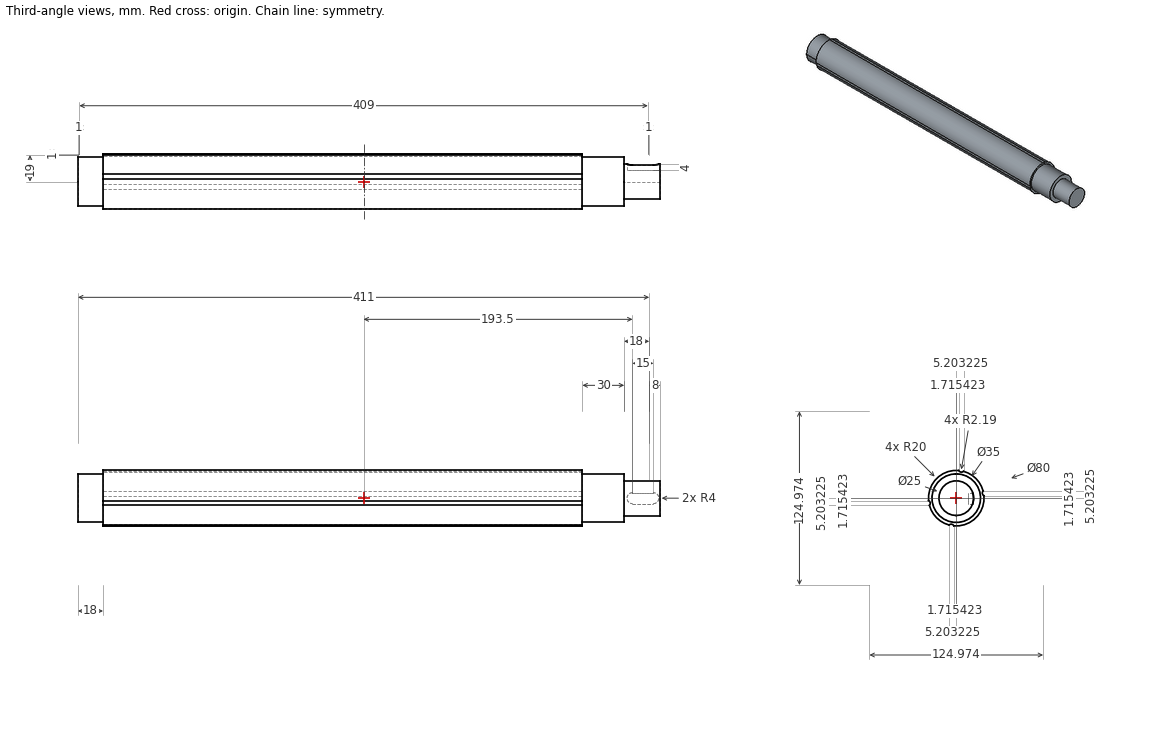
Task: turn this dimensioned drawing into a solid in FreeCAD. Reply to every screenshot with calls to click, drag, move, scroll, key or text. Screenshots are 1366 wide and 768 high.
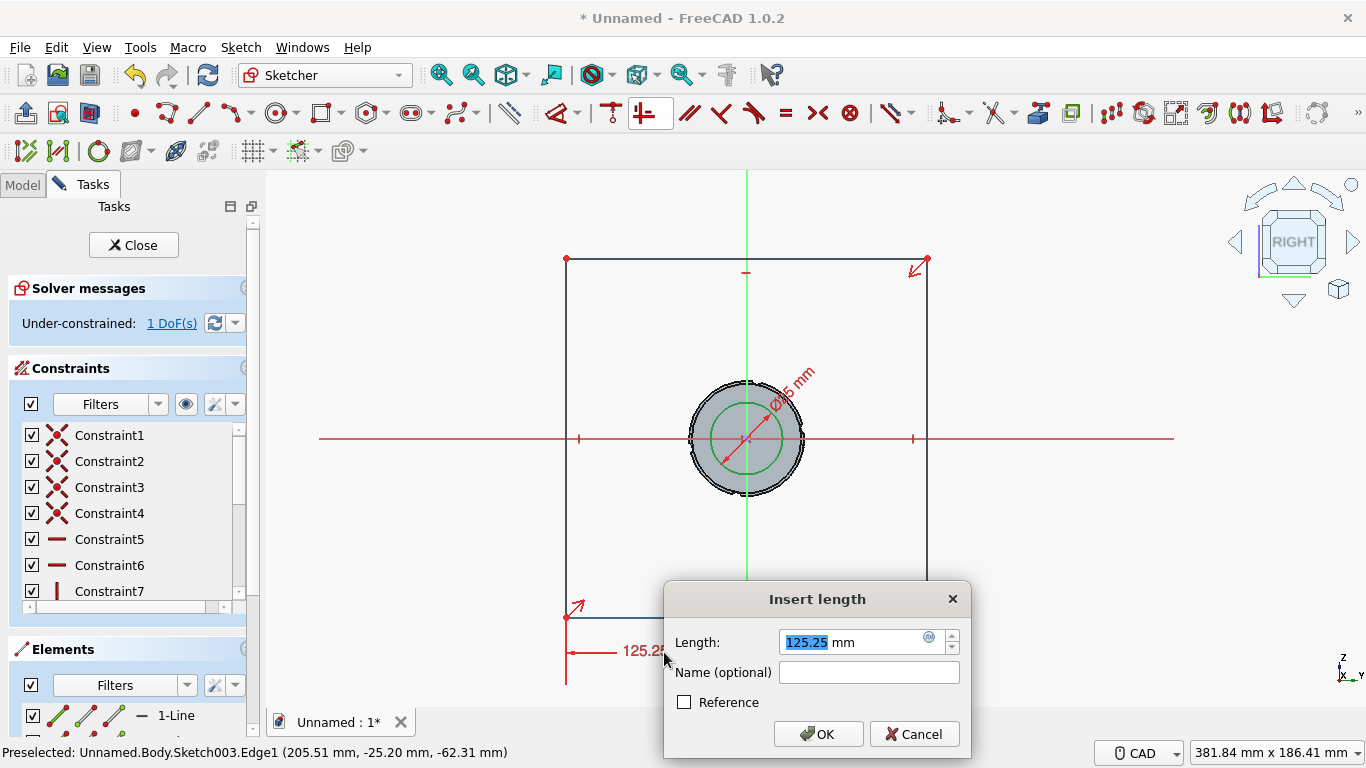
text(124.974)
key(Return)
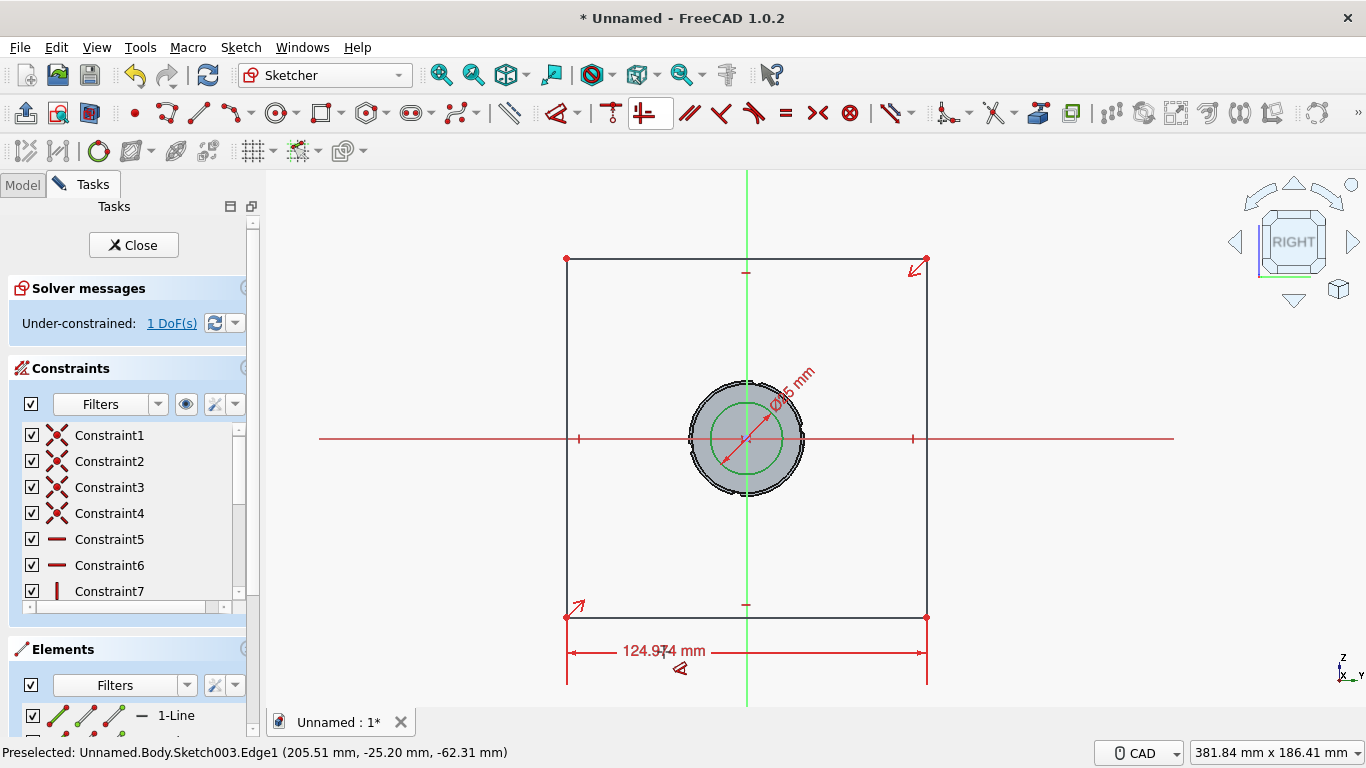
click(927, 510)
click(961, 356)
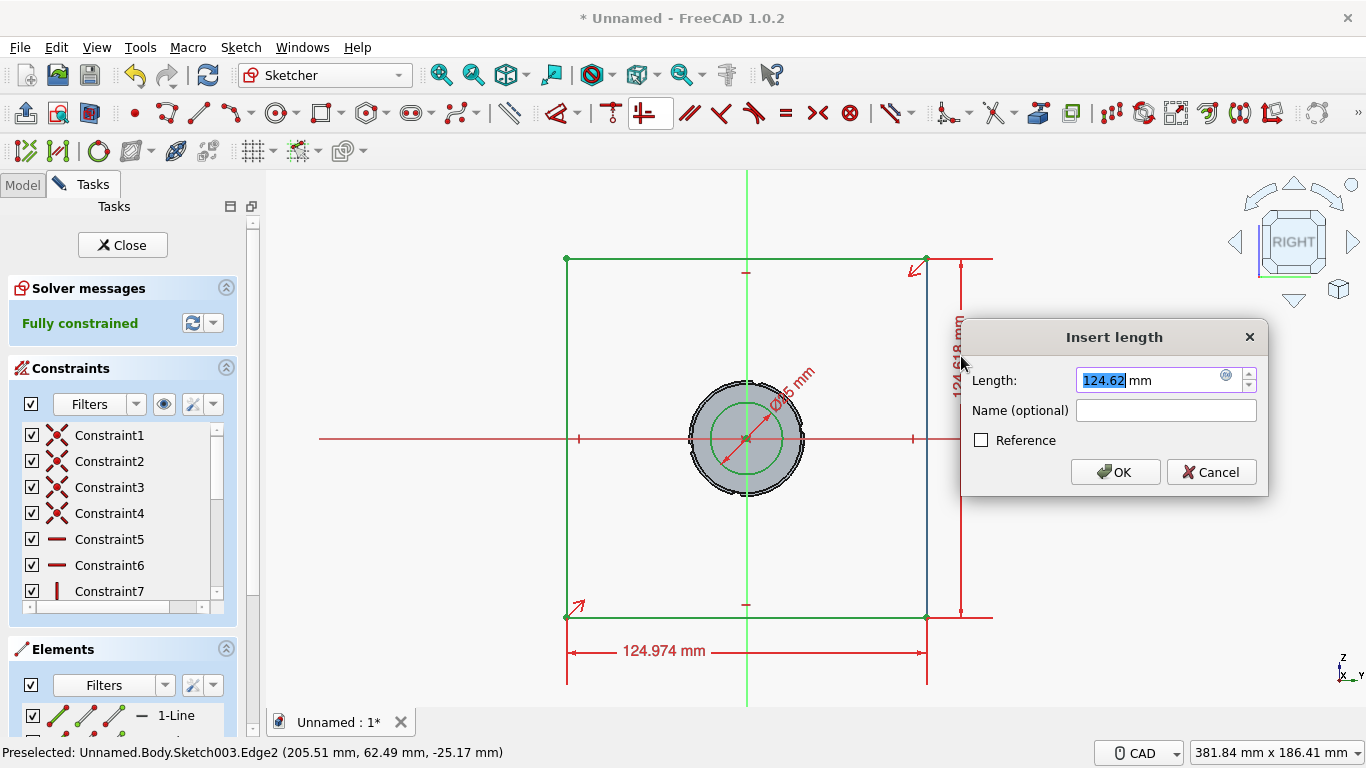
text(124.974)
key(Return)
key(Escape)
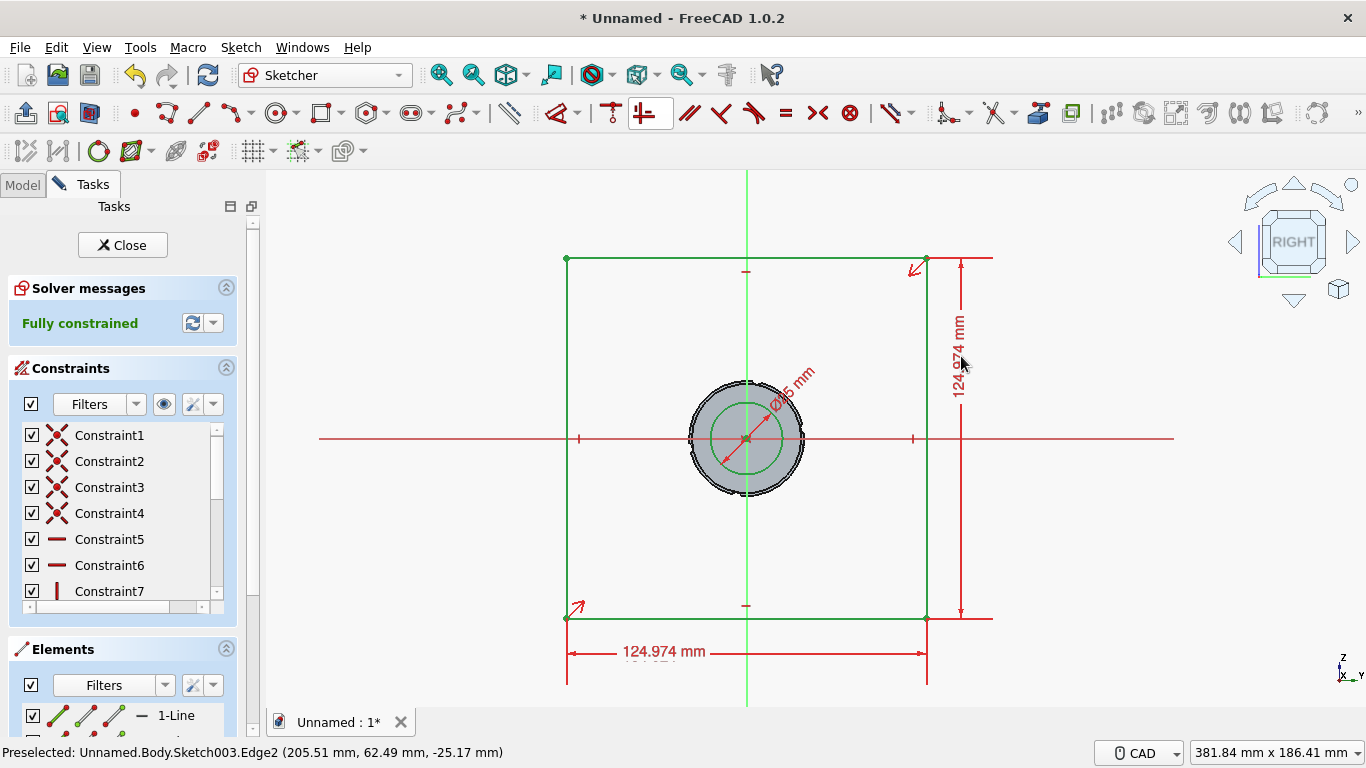
click(123, 245)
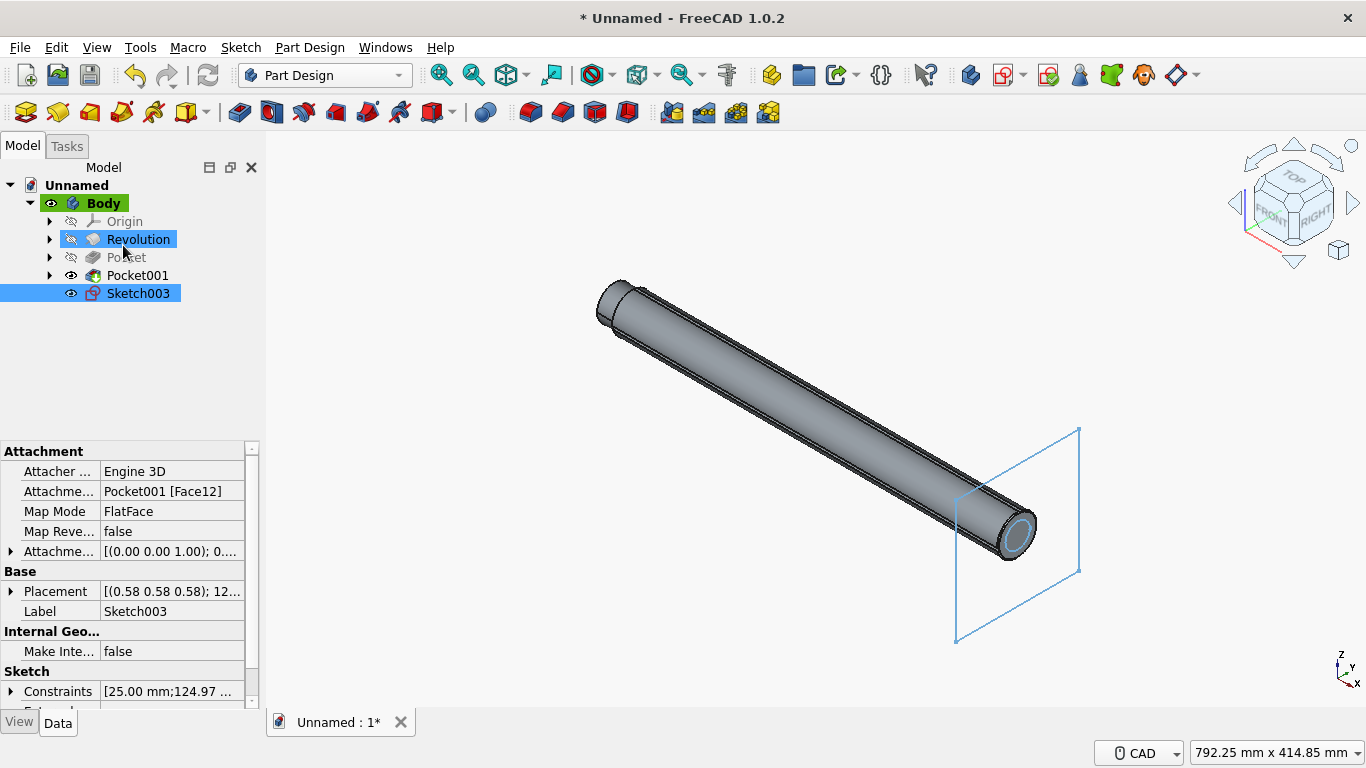
click(240, 112)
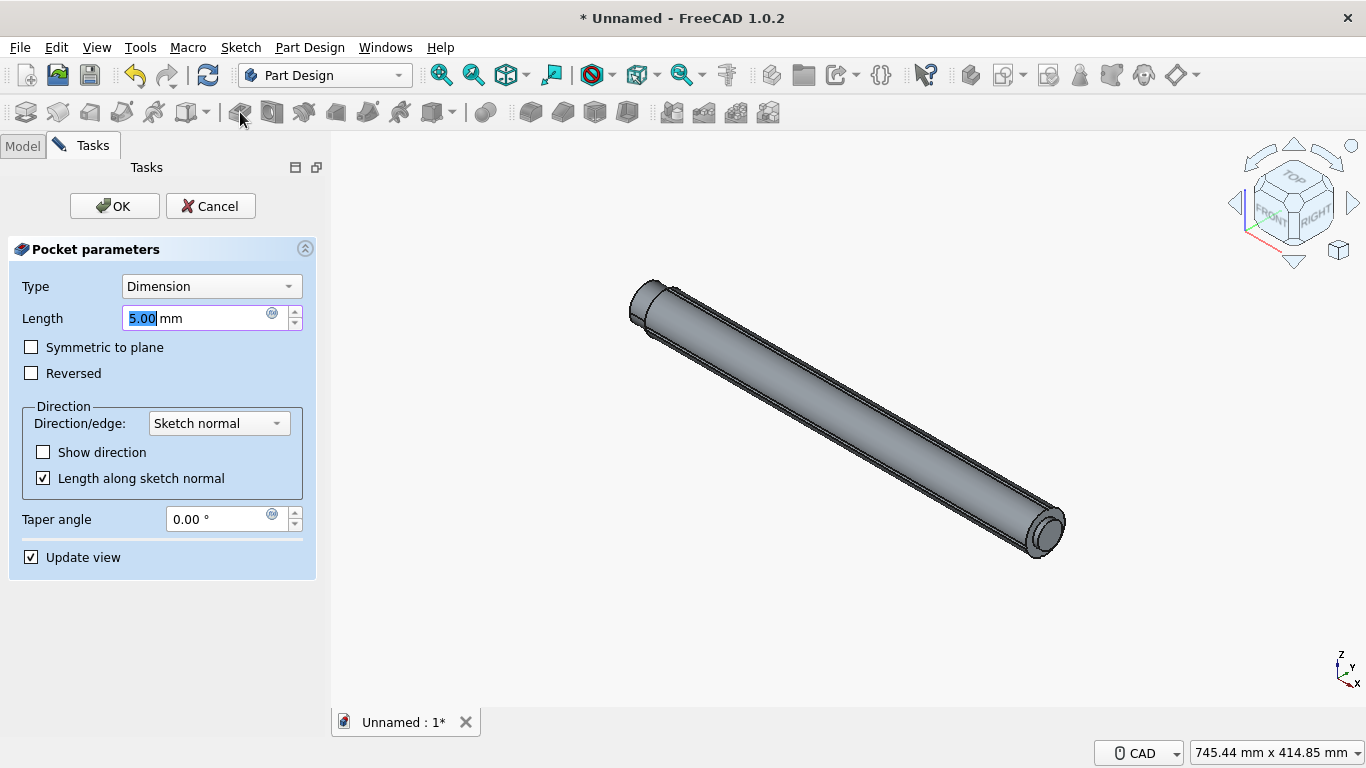
text(18)
key(Tab)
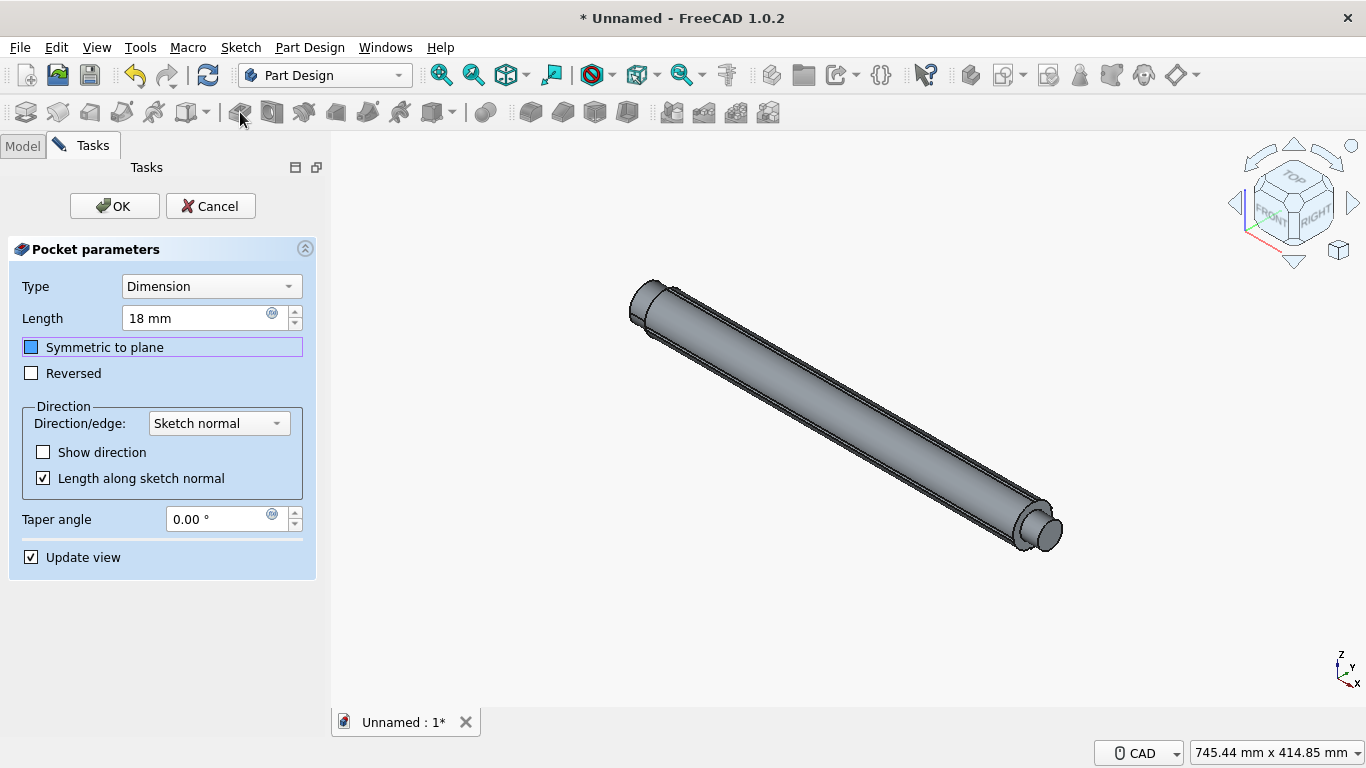
click(115, 206)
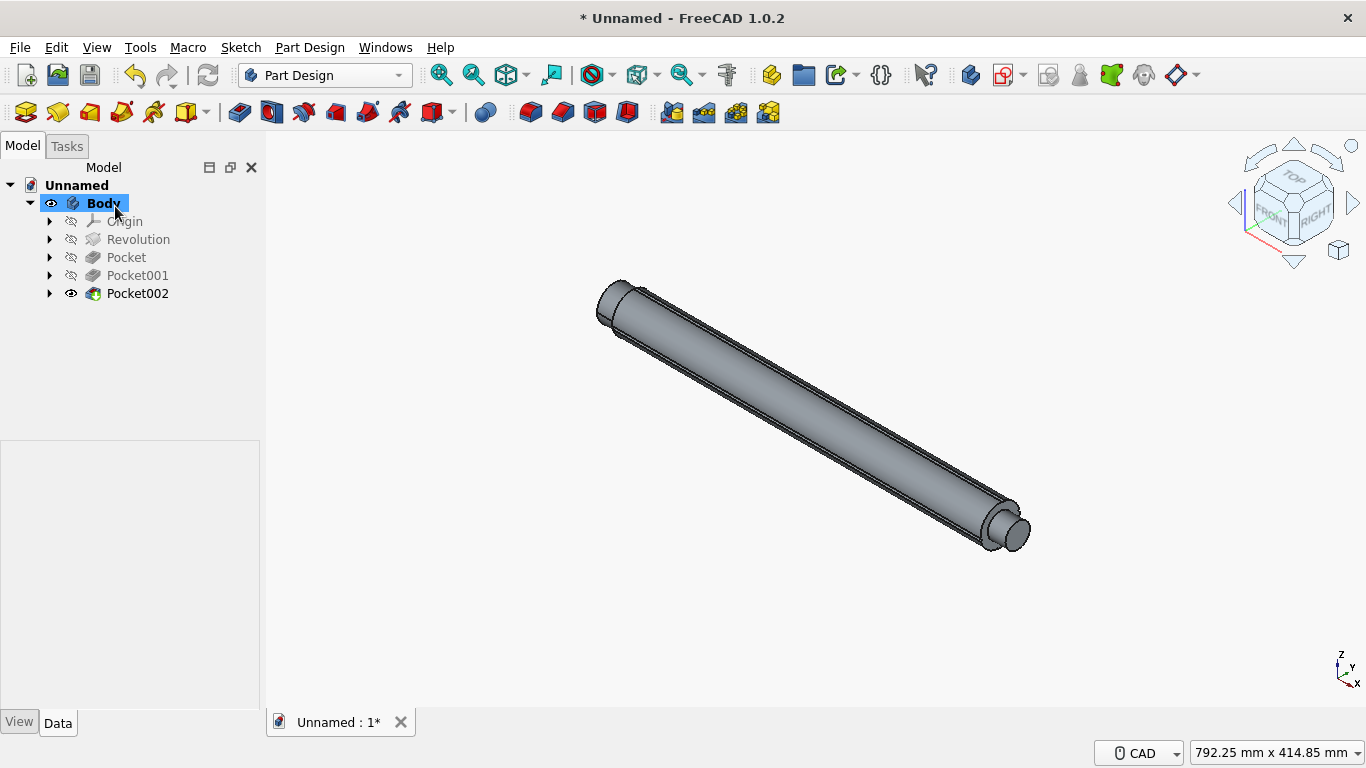
scroll(989, 518, up, 5)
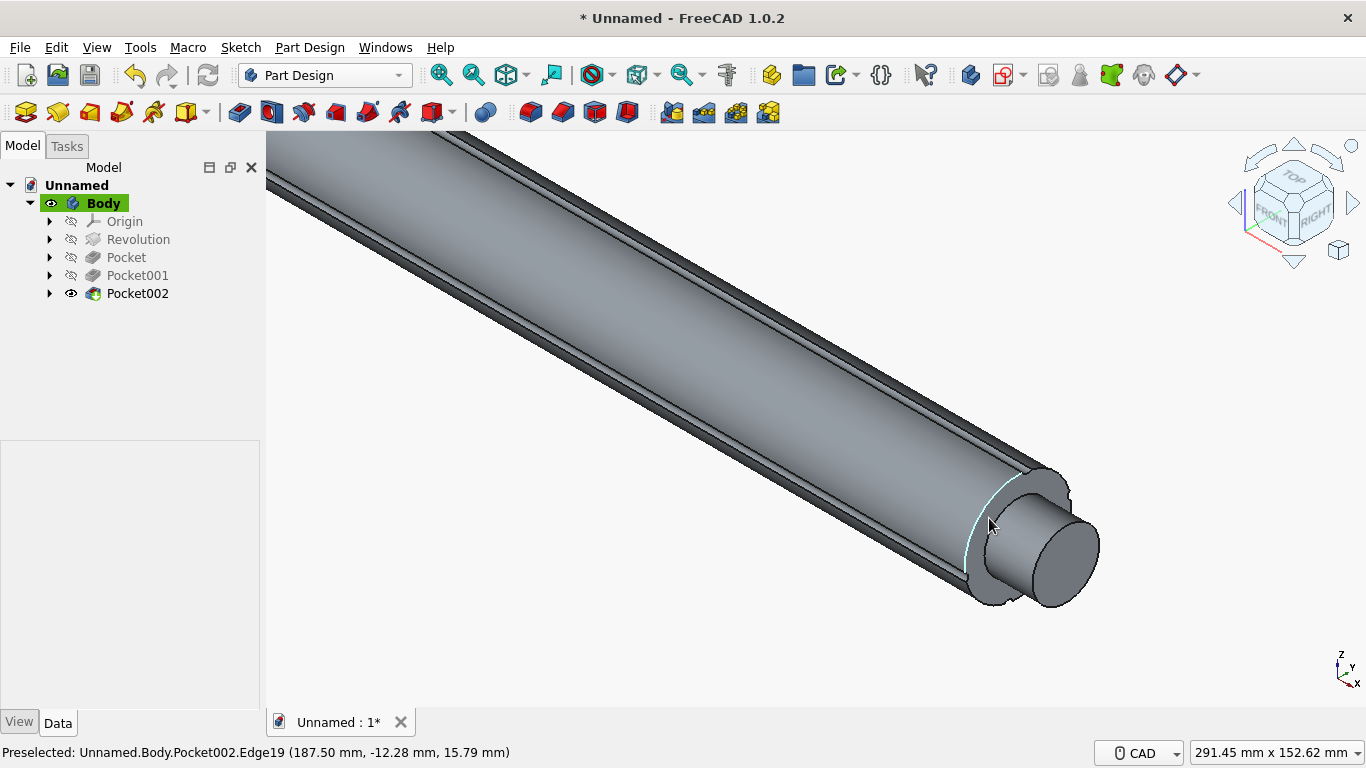
click(1048, 483)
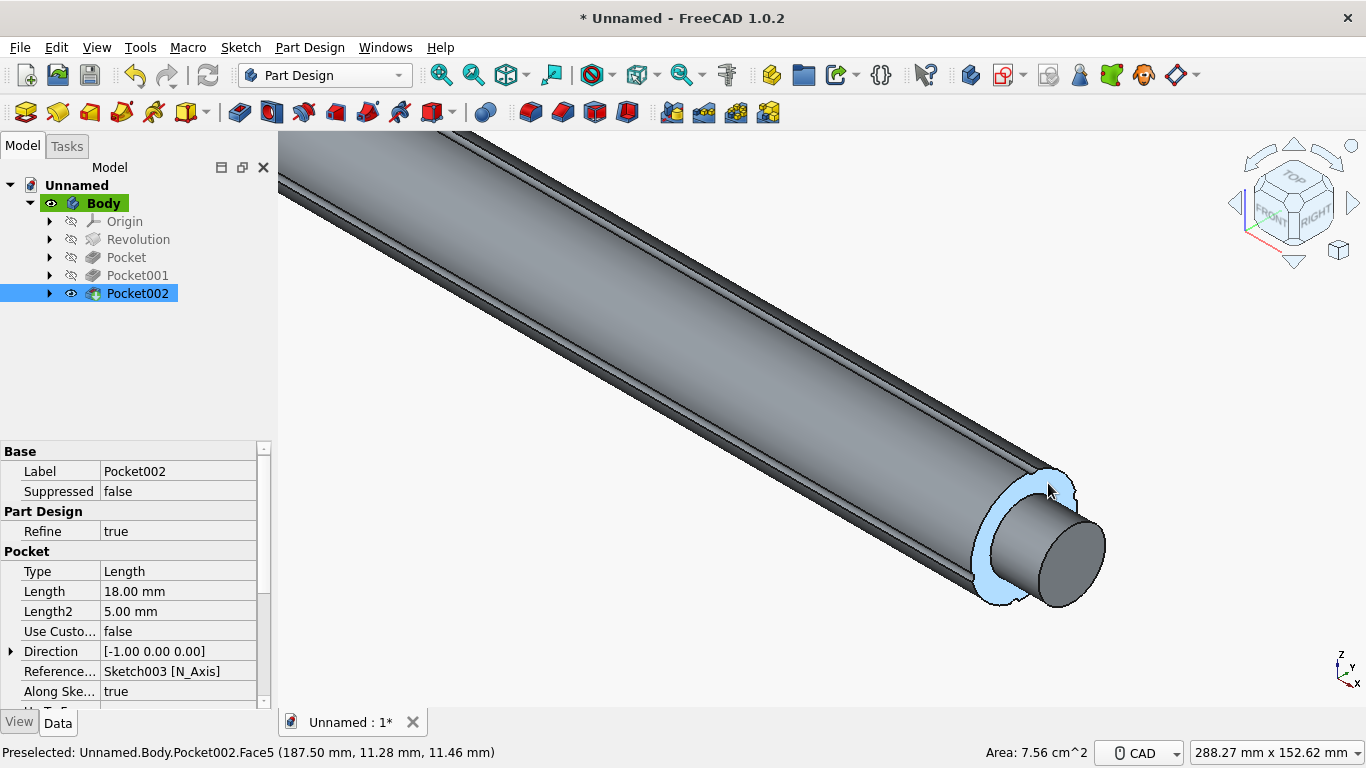
click(1004, 76)